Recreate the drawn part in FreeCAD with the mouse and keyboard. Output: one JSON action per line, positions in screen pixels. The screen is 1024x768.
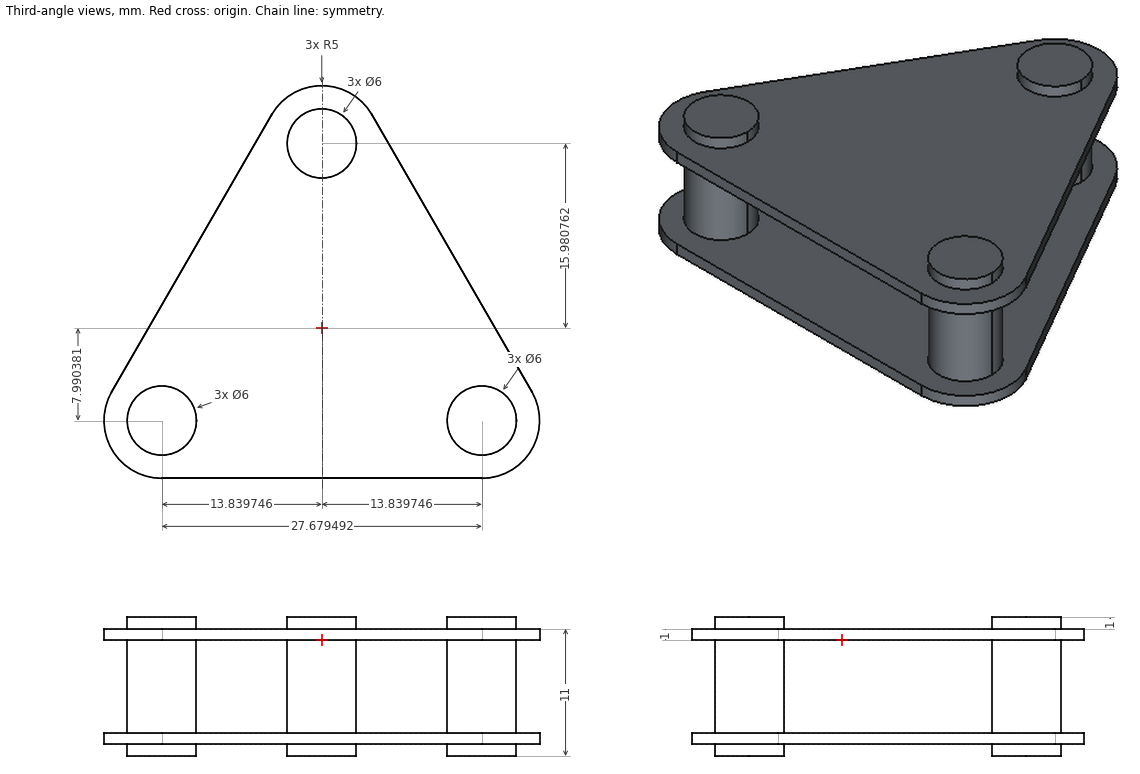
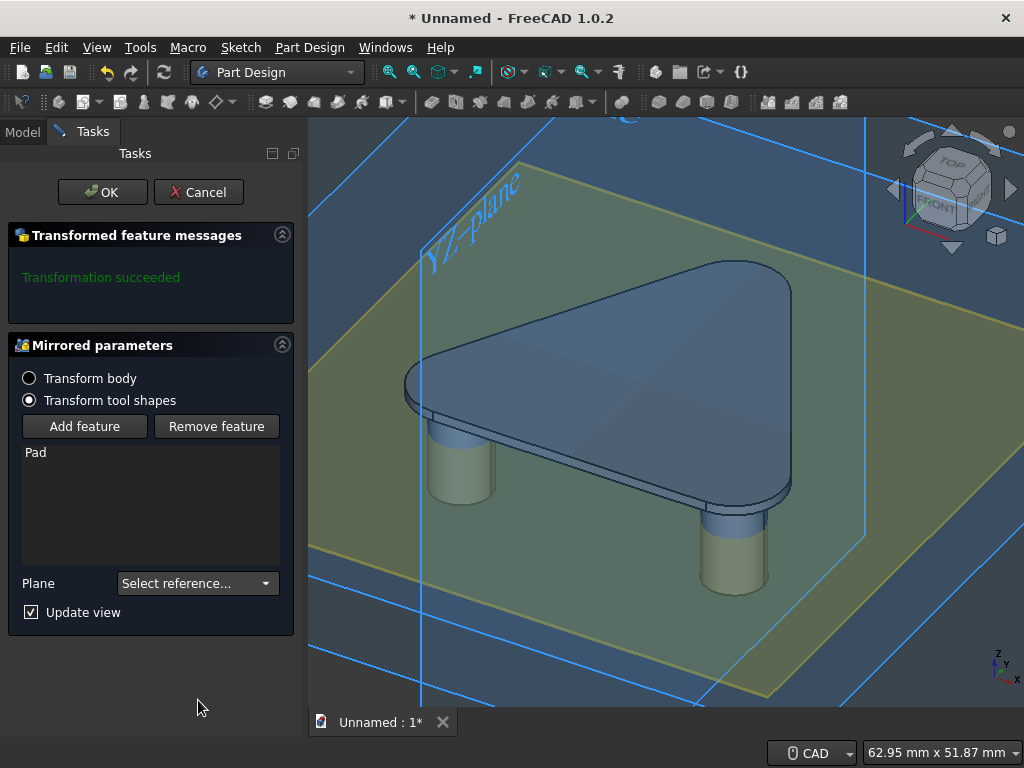
{"action": "left_click", "coordinate": [23, 131]}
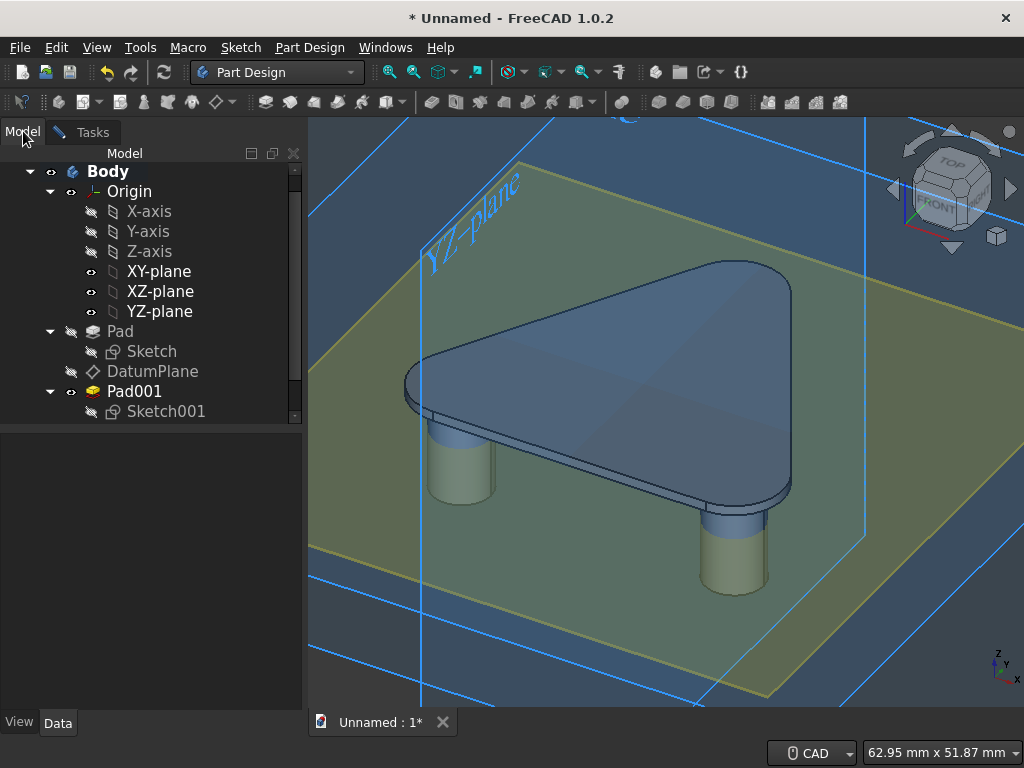
{"action": "scroll", "coordinate": [120, 287], "scroll_direction": "down", "scroll_amount": 3}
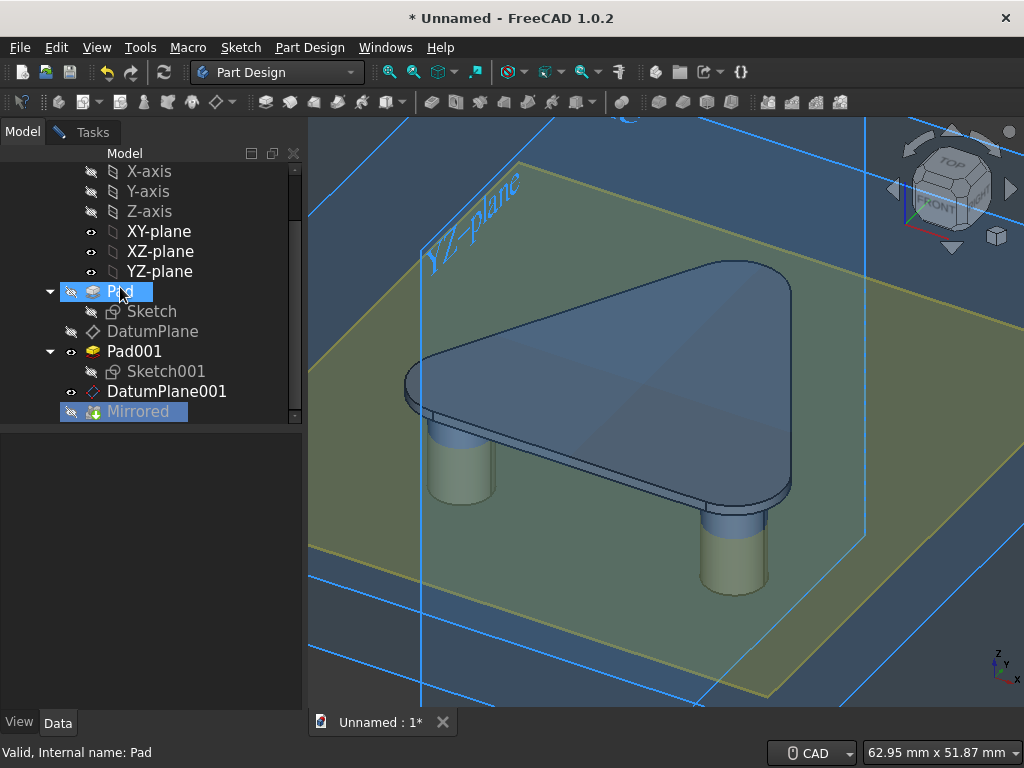
{"action": "left_click", "coordinate": [116, 392]}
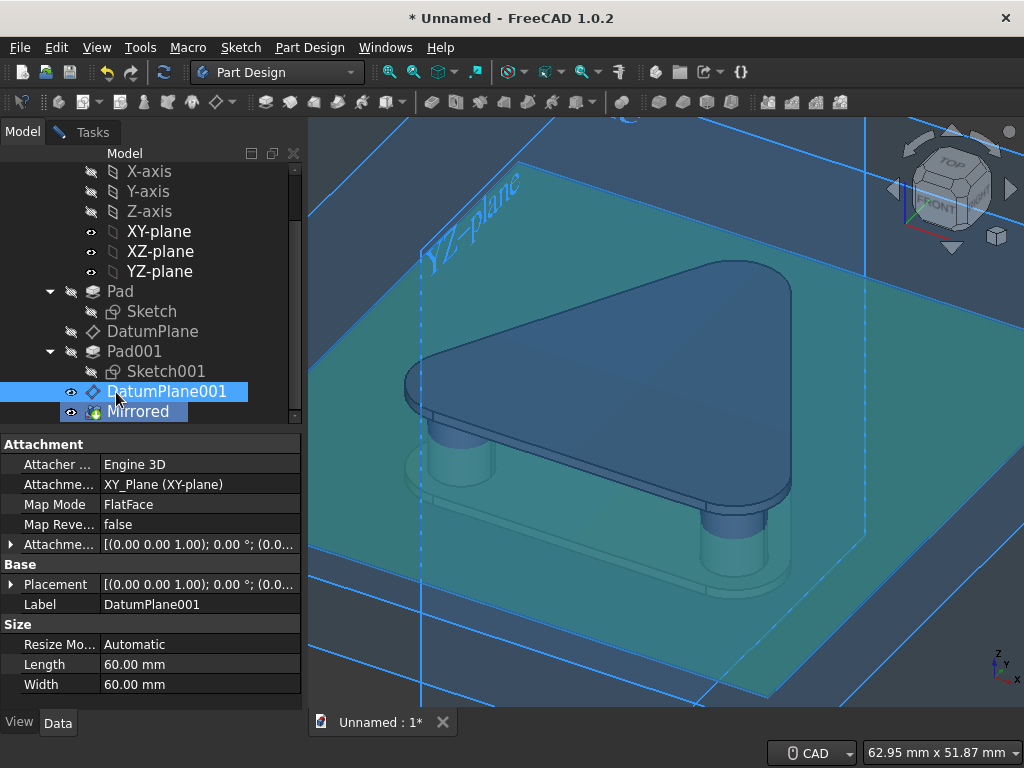
{"action": "left_click", "coordinate": [84, 131]}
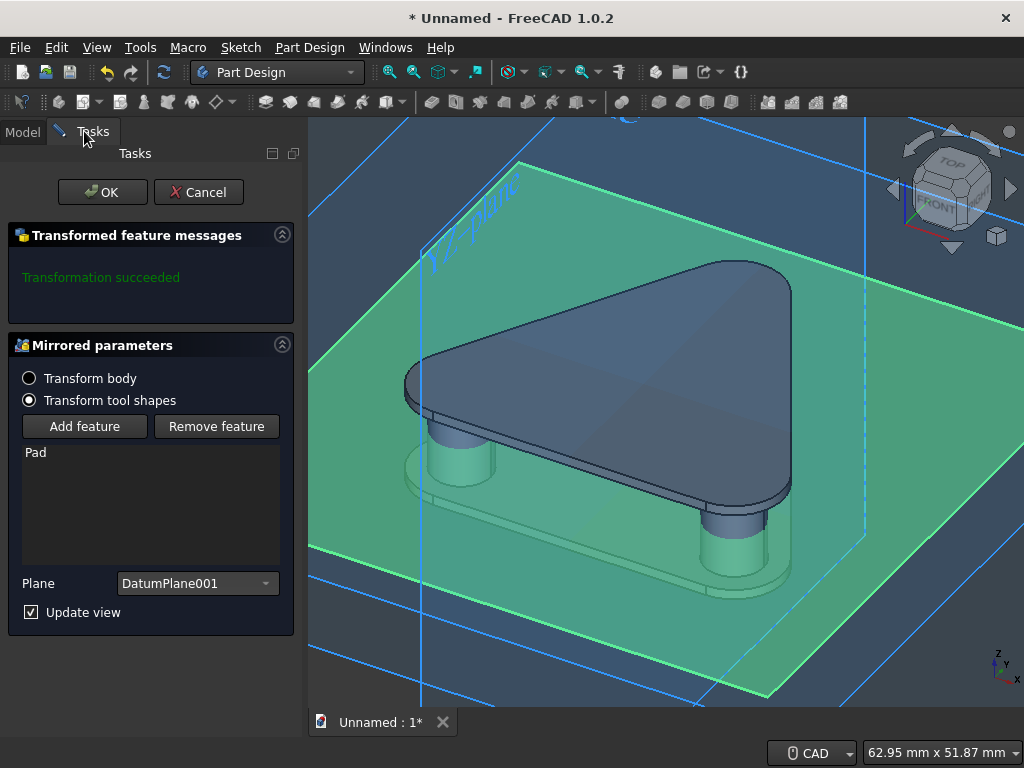
{"action": "left_click", "coordinate": [103, 192]}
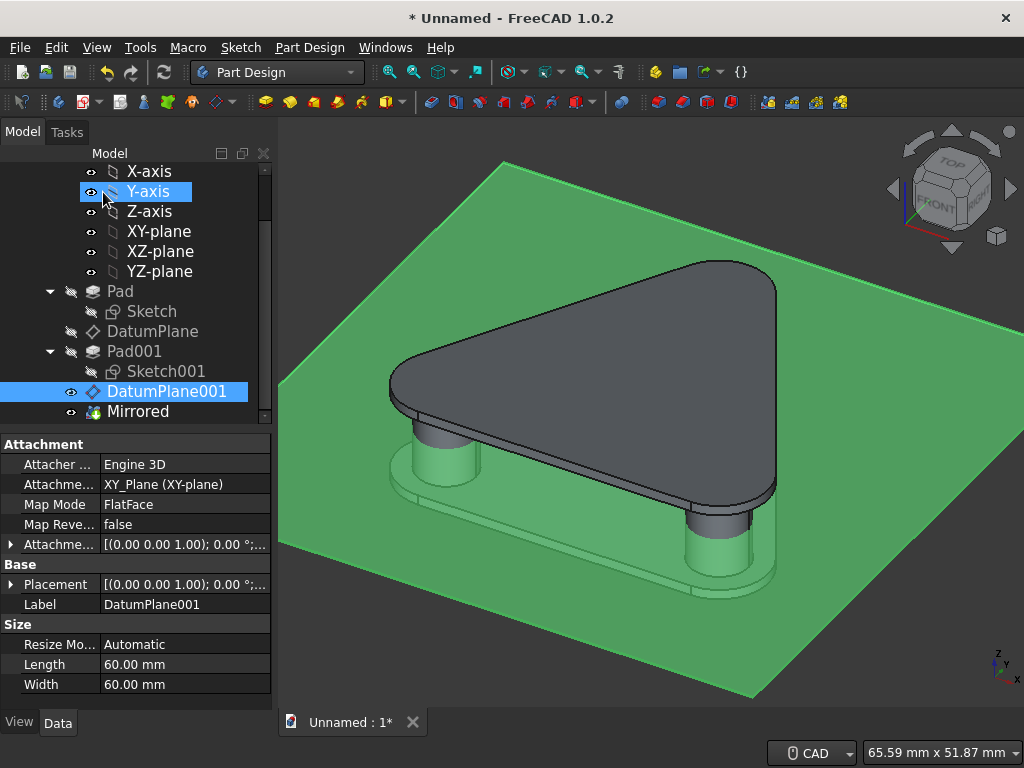
{"action": "left_click", "coordinate": [116, 392]}
{"action": "key", "text": "space"}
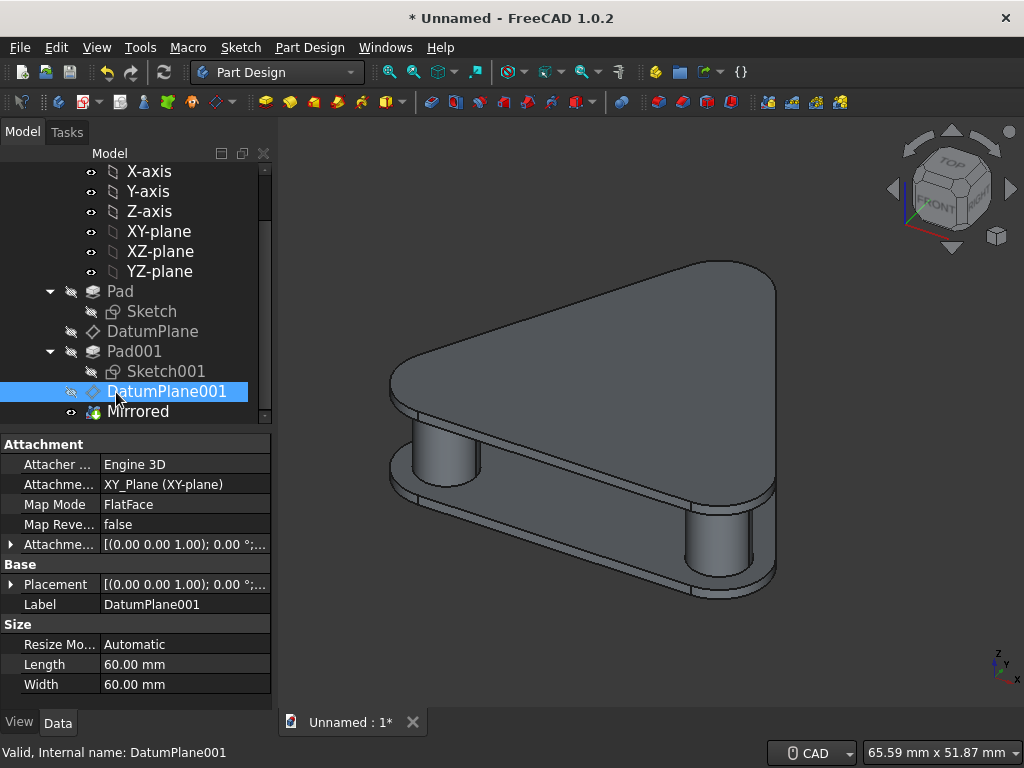
{"action": "left_click", "coordinate": [623, 387]}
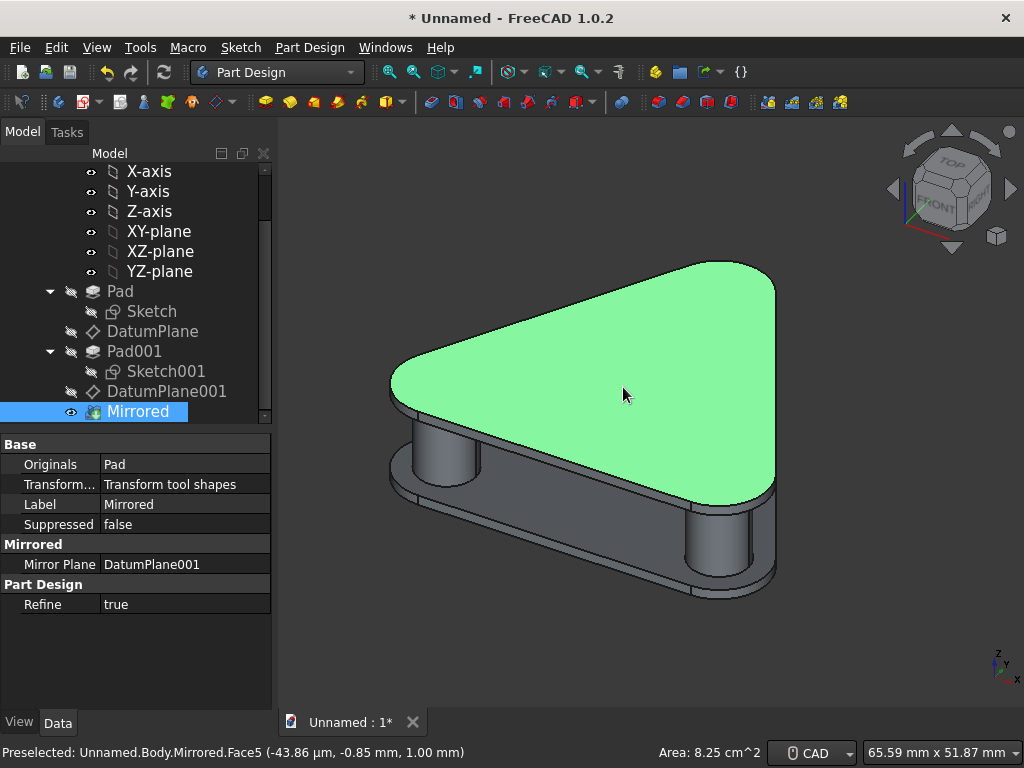
{"action": "left_click", "coordinate": [84, 102]}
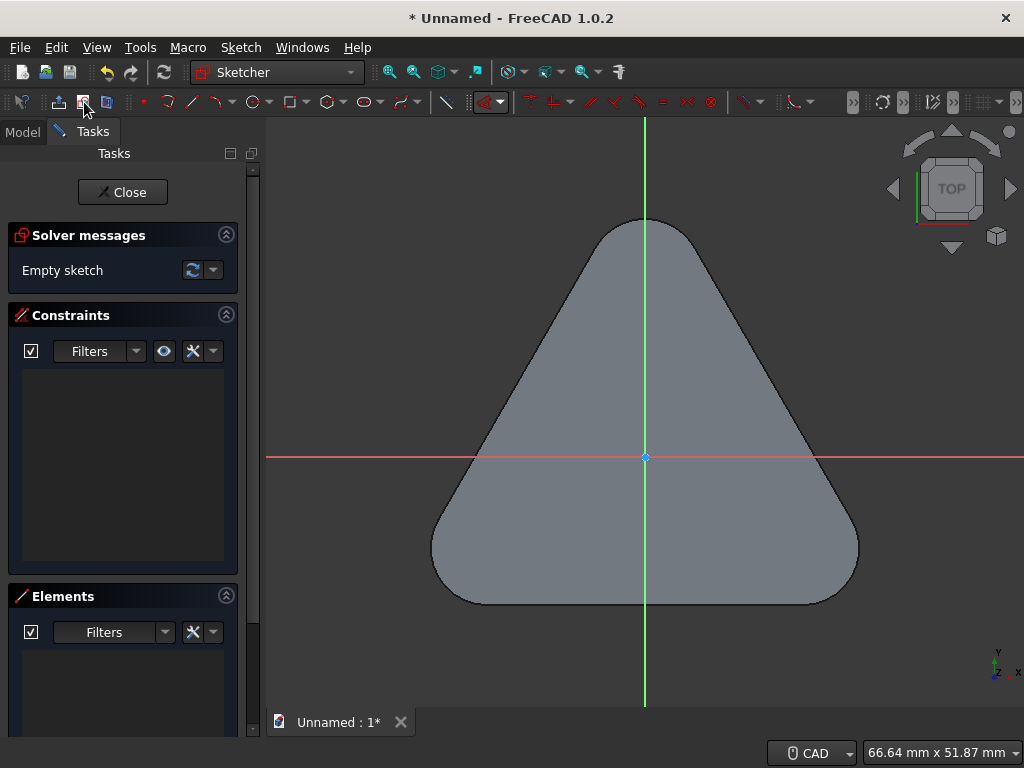
{"action": "scroll", "coordinate": [294, 412], "scroll_direction": "down", "scroll_amount": 1}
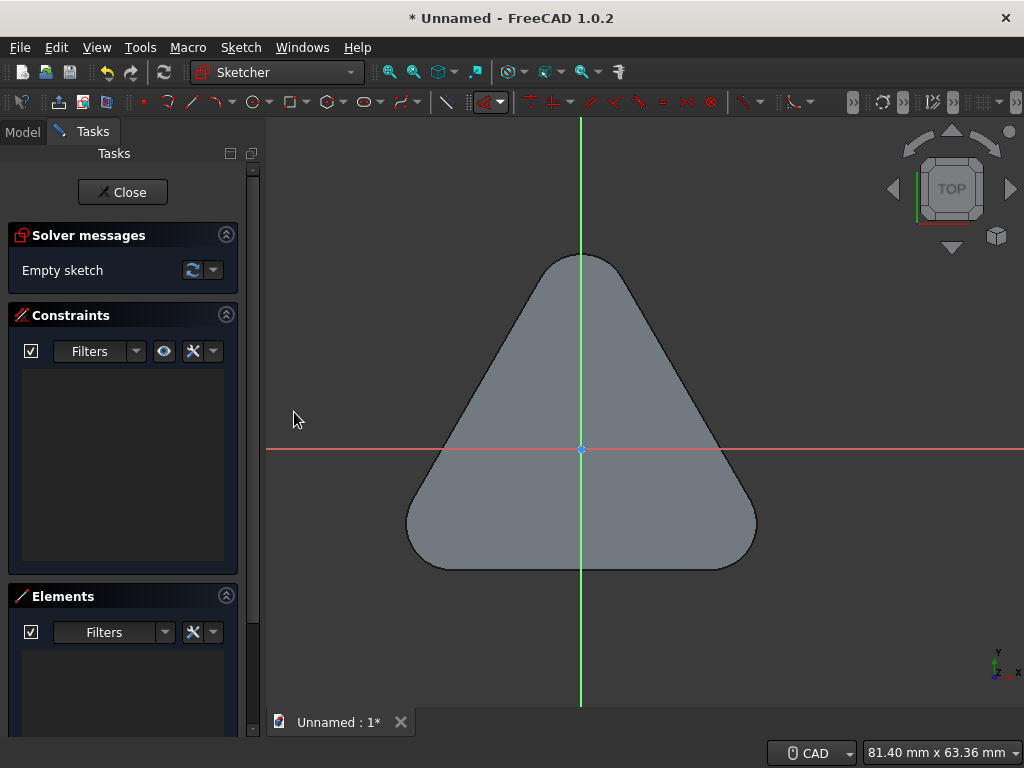
{"action": "left_click", "coordinate": [254, 102]}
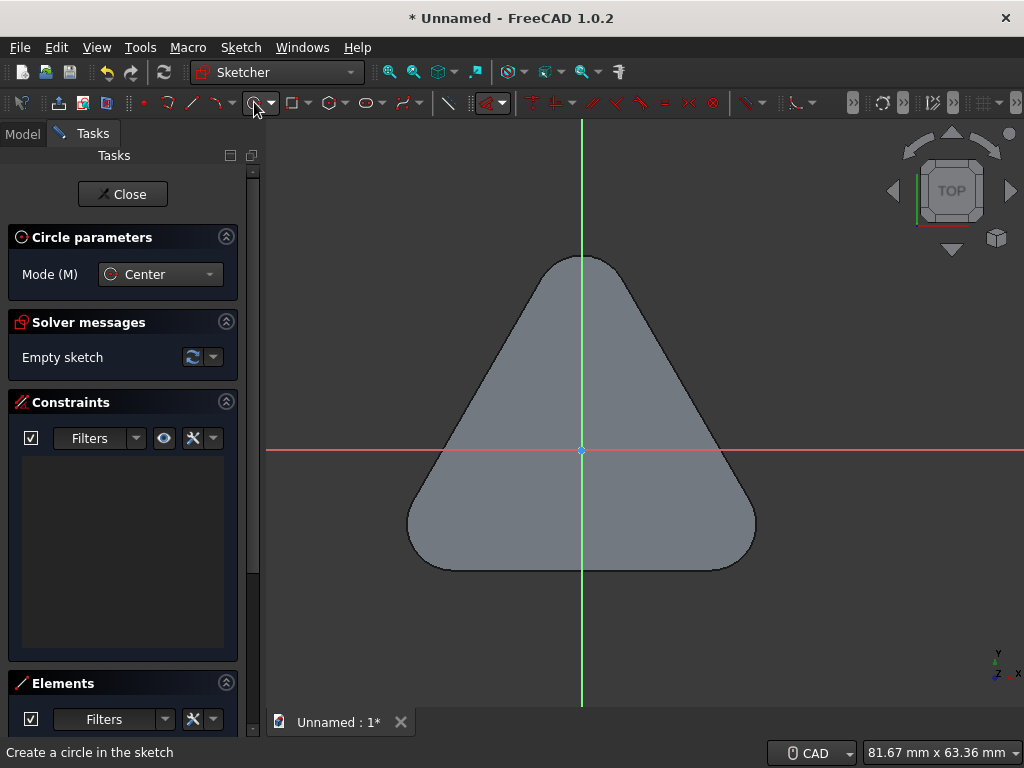
{"action": "left_click", "coordinate": [582, 302]}
{"action": "mouse_move", "coordinate": [601, 282]}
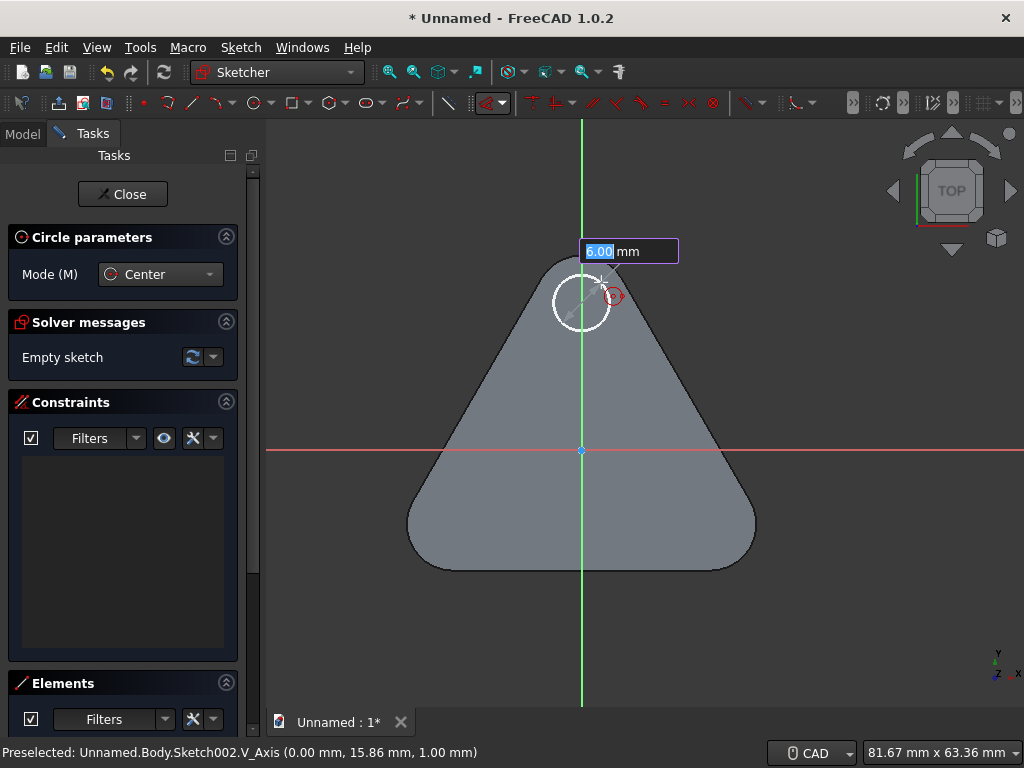
{"action": "type", "text": "6"}
{"action": "key", "text": "Return"}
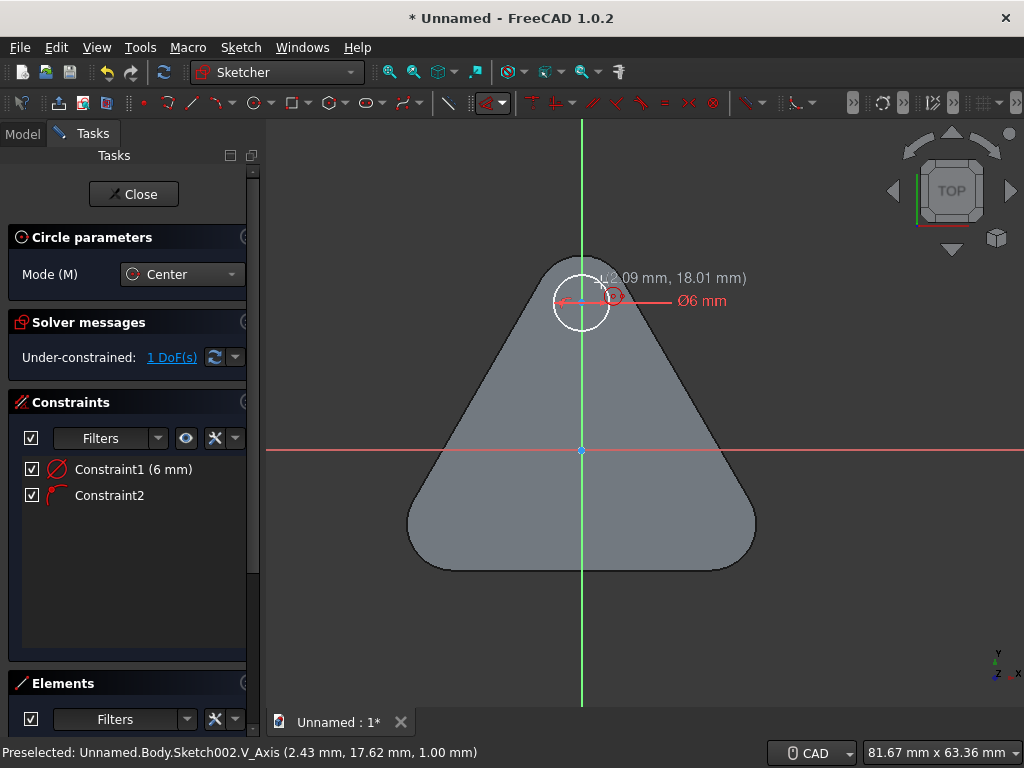
{"action": "left_click", "coordinate": [710, 524]}
{"action": "mouse_move", "coordinate": [730, 505]}